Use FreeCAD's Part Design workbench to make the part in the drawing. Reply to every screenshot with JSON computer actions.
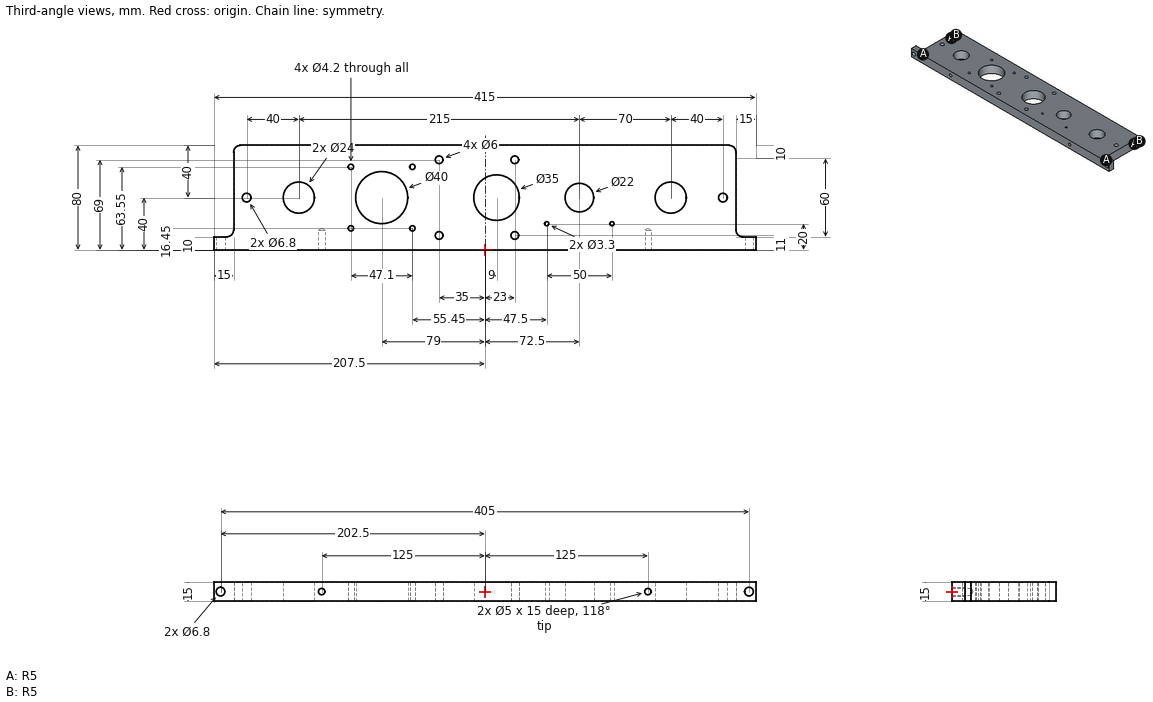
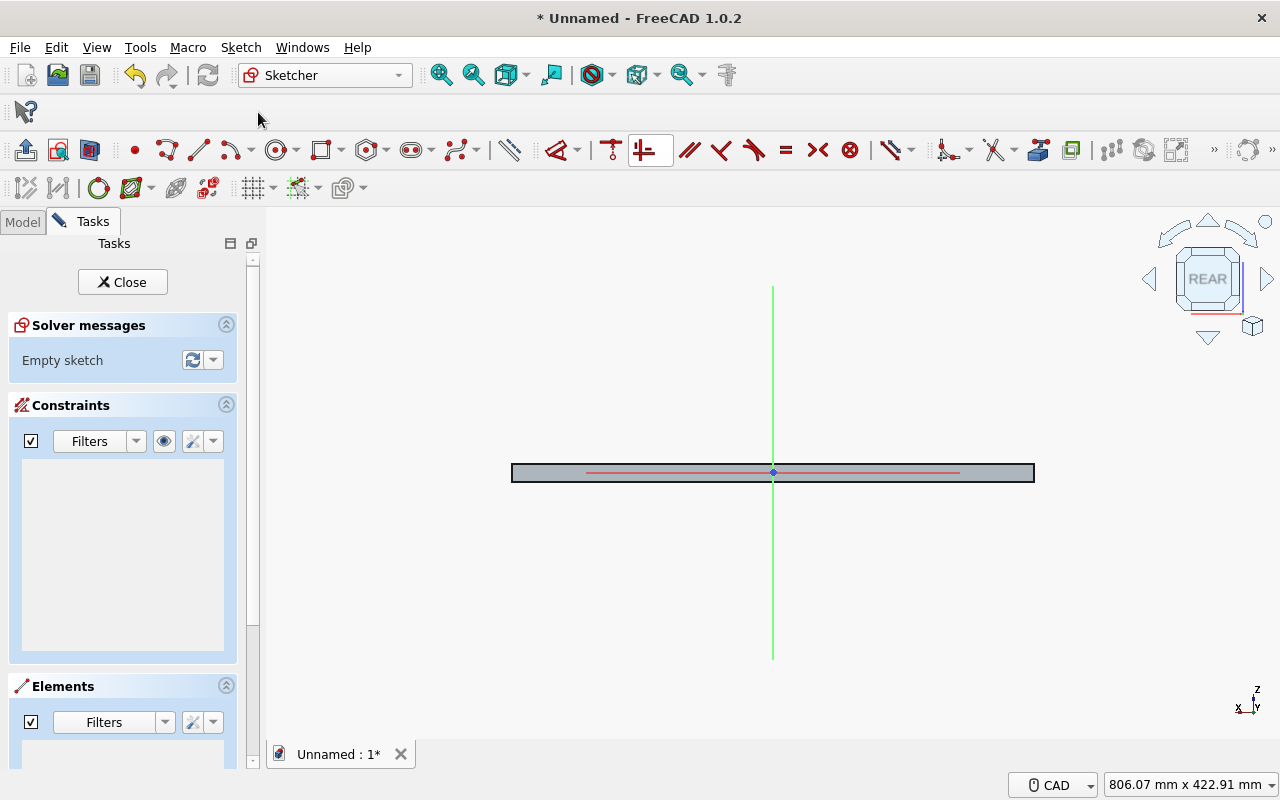
{"action": "left_click", "coordinate": [276, 150]}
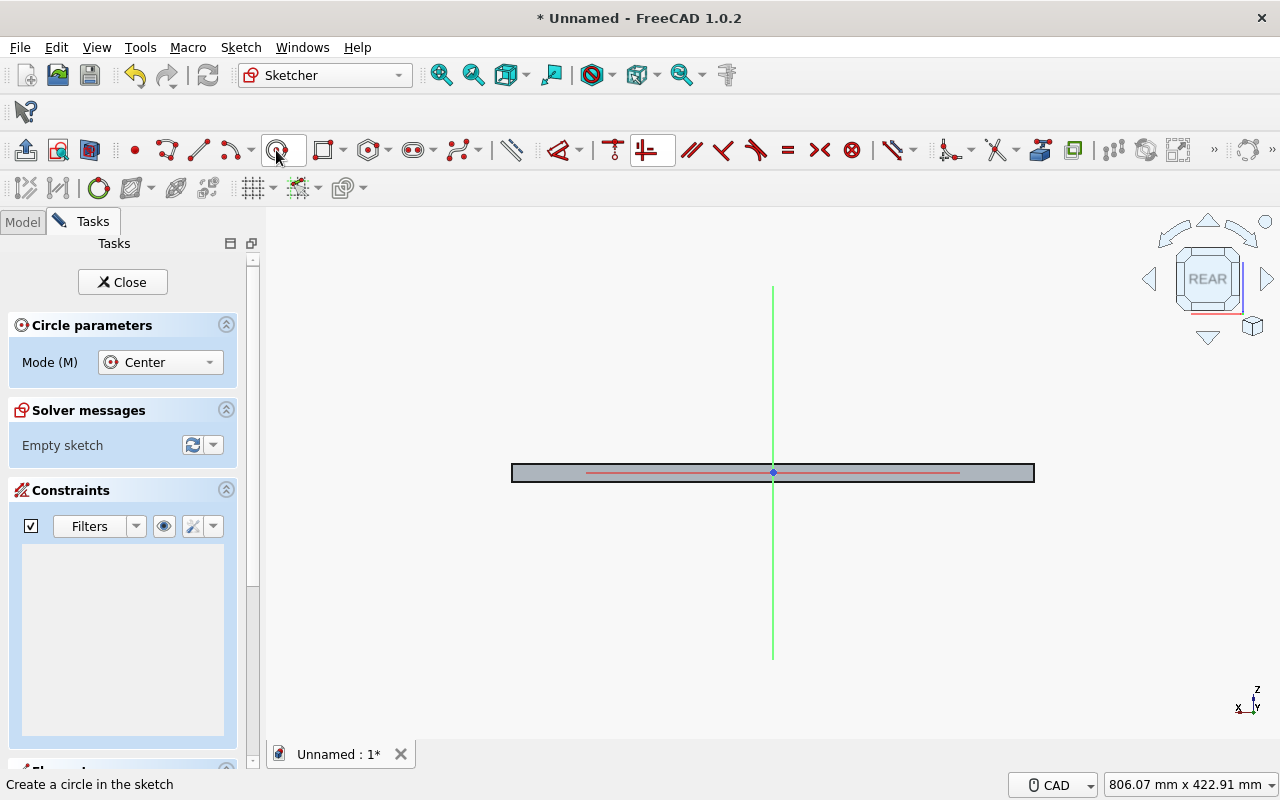
{"action": "scroll", "coordinate": [1028, 473], "scroll_direction": "up", "scroll_amount": 9}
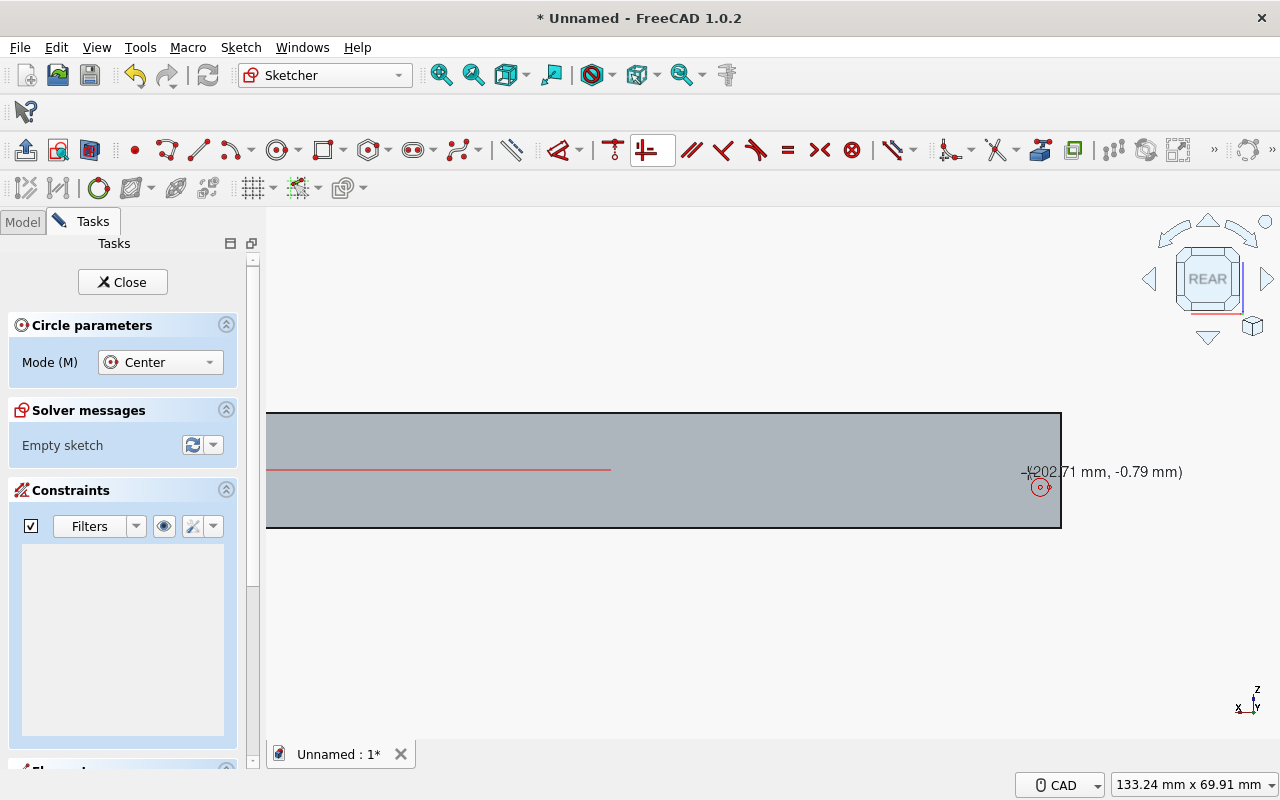
{"action": "scroll", "coordinate": [1014, 474], "scroll_direction": "down", "scroll_amount": 8}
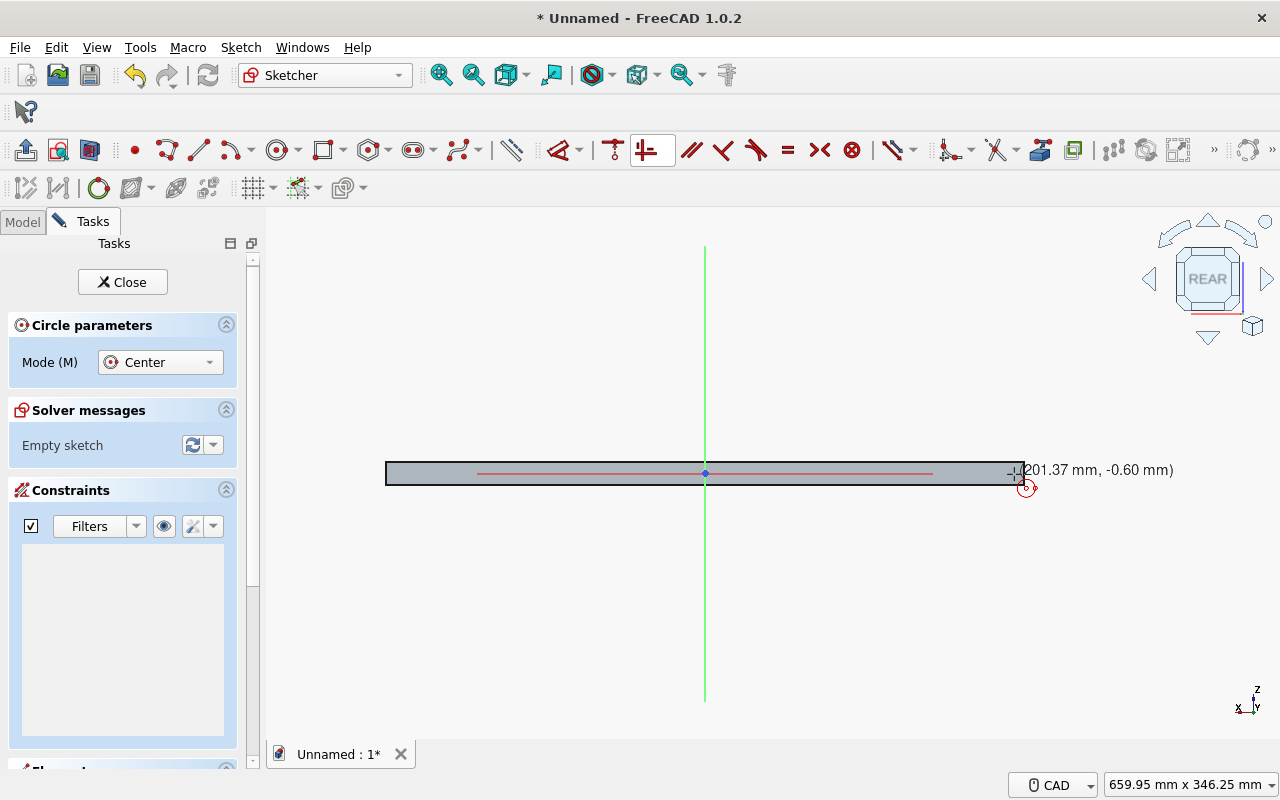
{"action": "left_click", "coordinate": [1016, 474]}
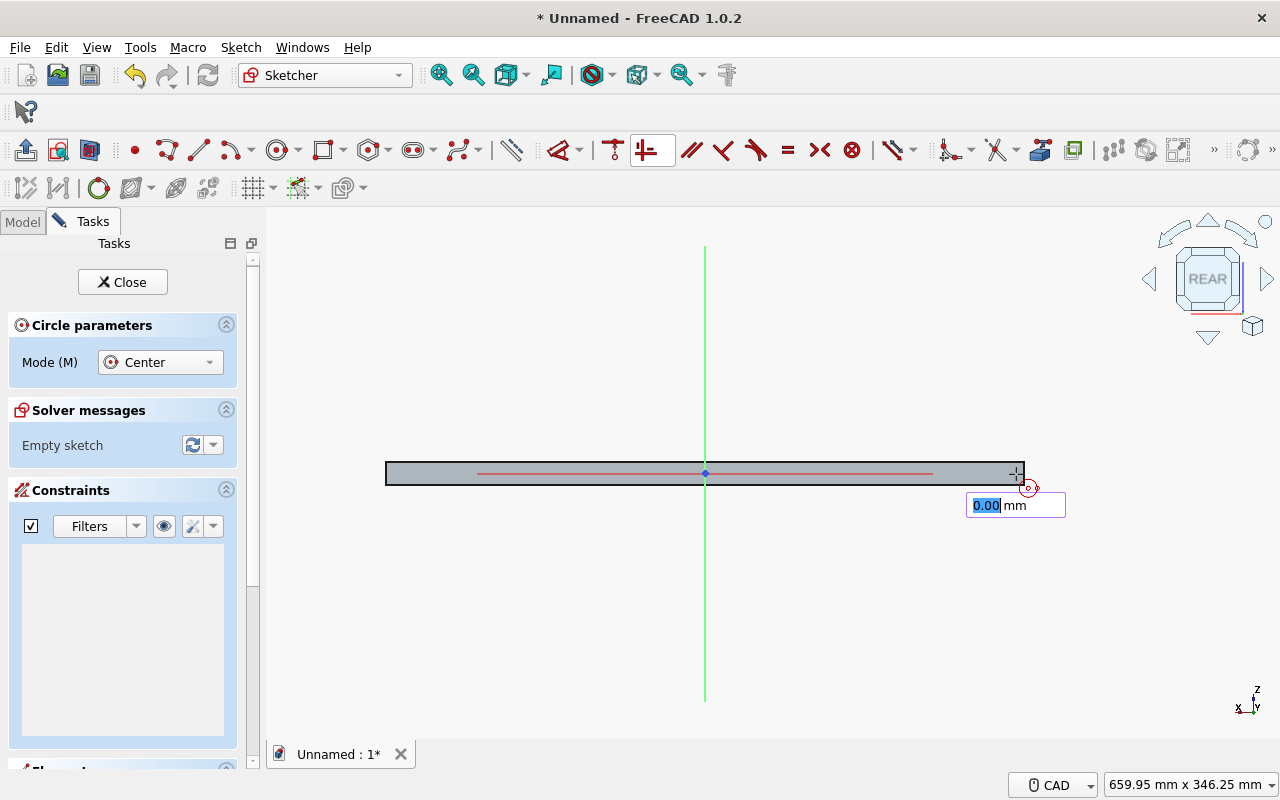
{"action": "scroll", "coordinate": [1015, 479], "scroll_direction": "up", "scroll_amount": 6}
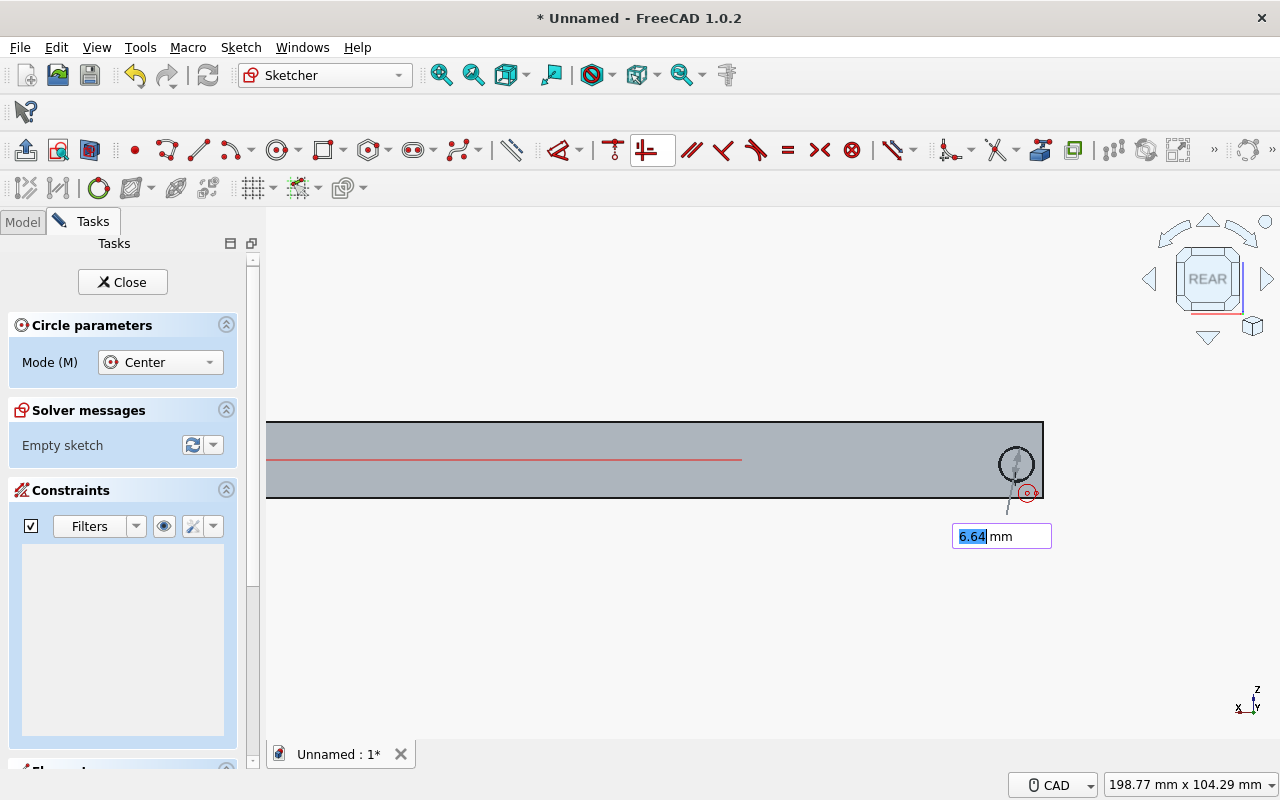
{"action": "left_click", "coordinate": [1012, 476]}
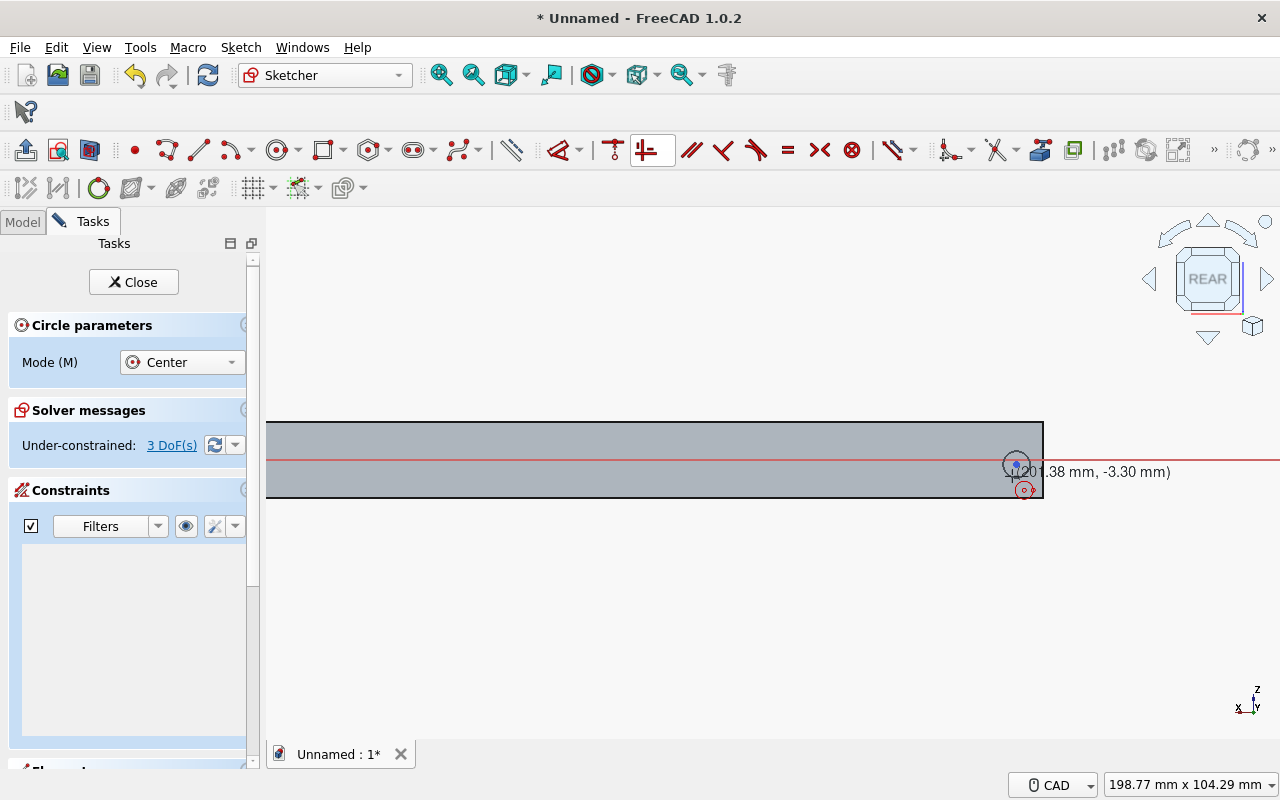
{"action": "scroll", "coordinate": [1015, 479], "scroll_direction": "down", "scroll_amount": 6}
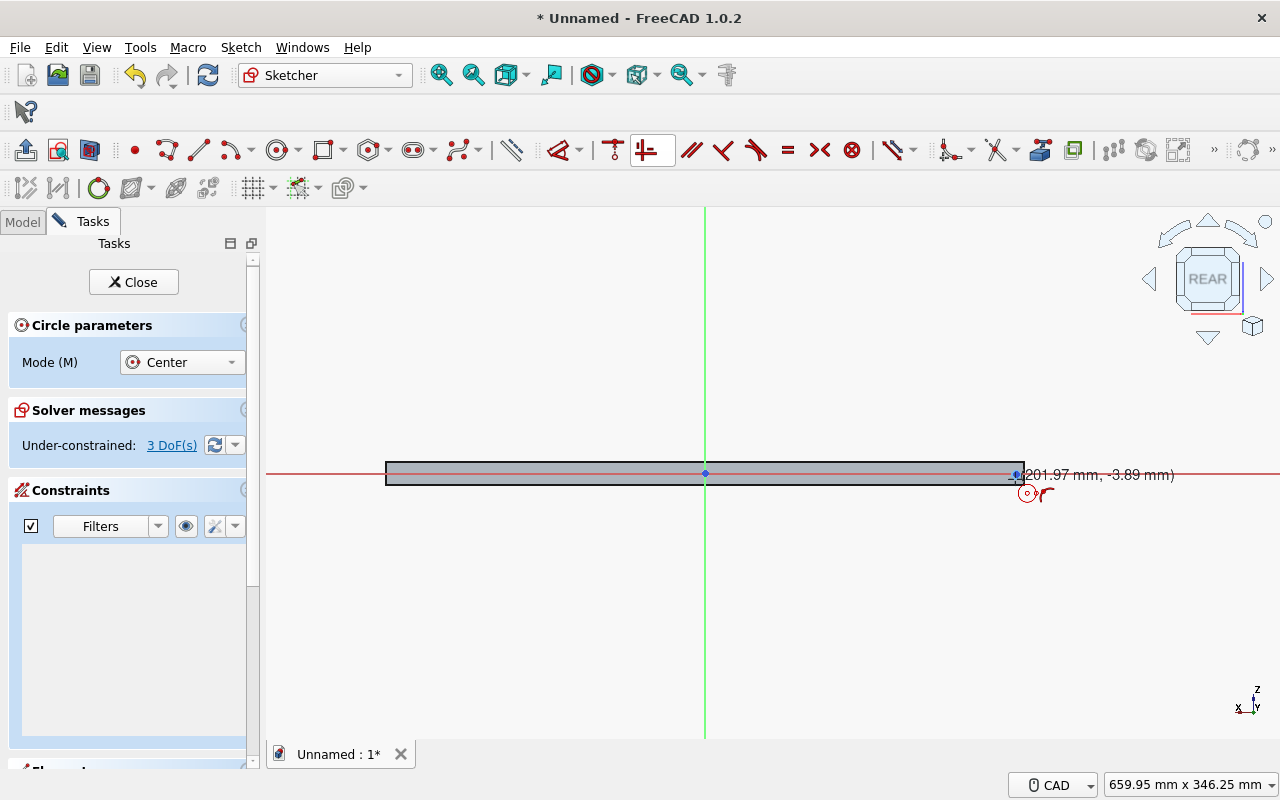
{"action": "scroll", "coordinate": [394, 474], "scroll_direction": "up", "scroll_amount": 8}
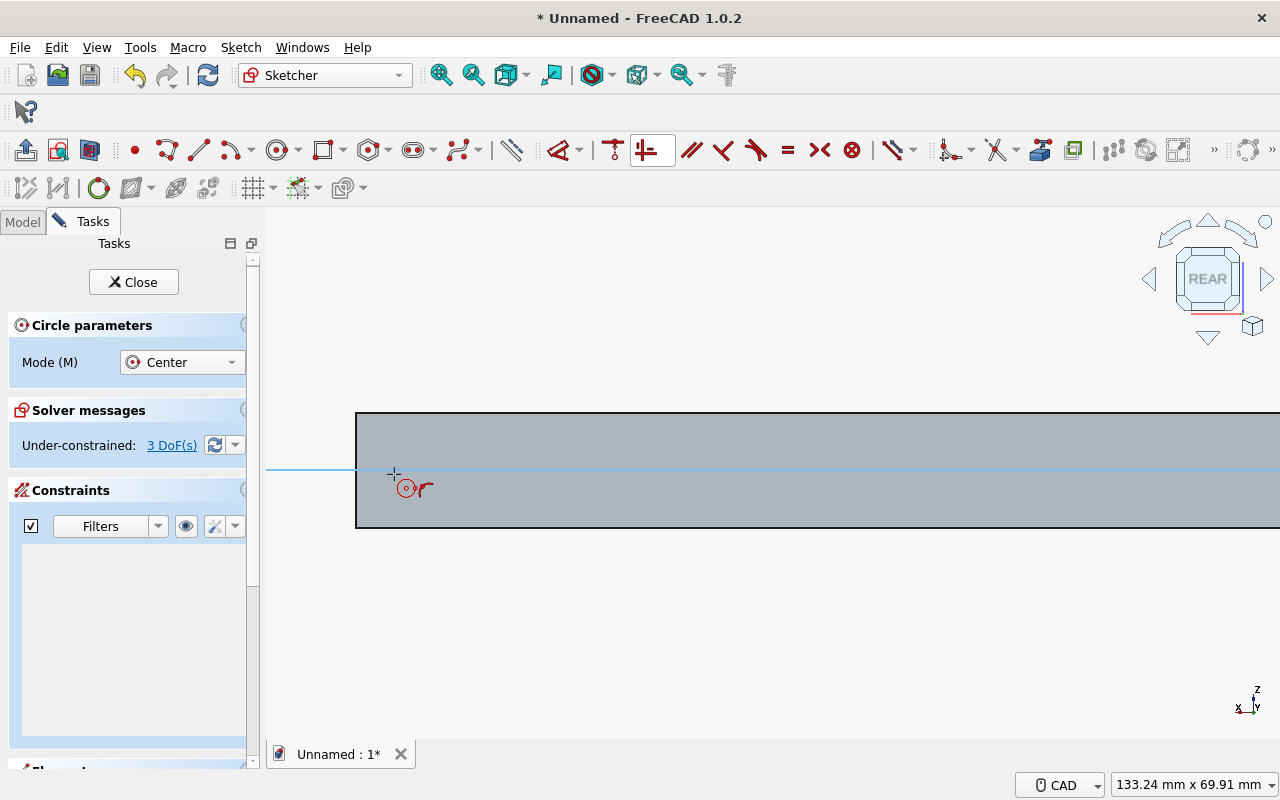
{"action": "scroll", "coordinate": [393, 474], "scroll_direction": "down", "scroll_amount": 8}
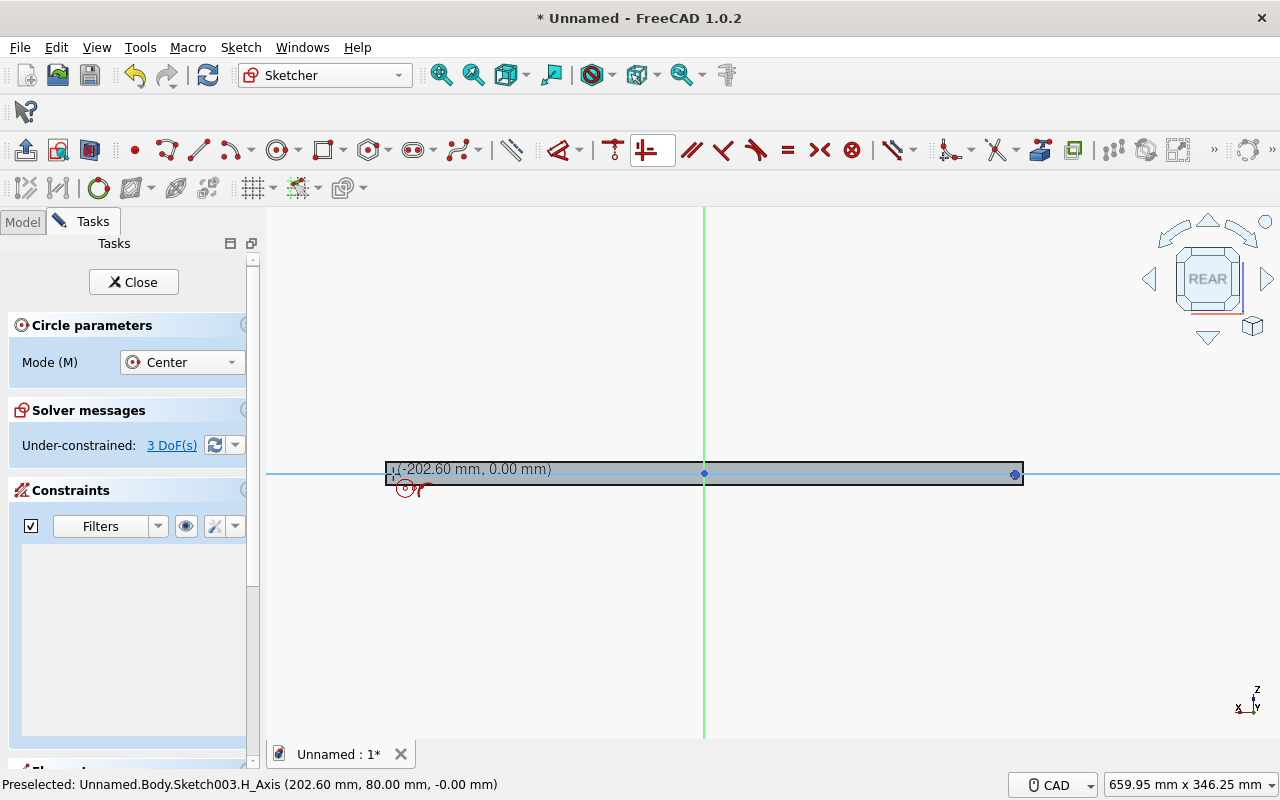
{"action": "left_click", "coordinate": [393, 474]}